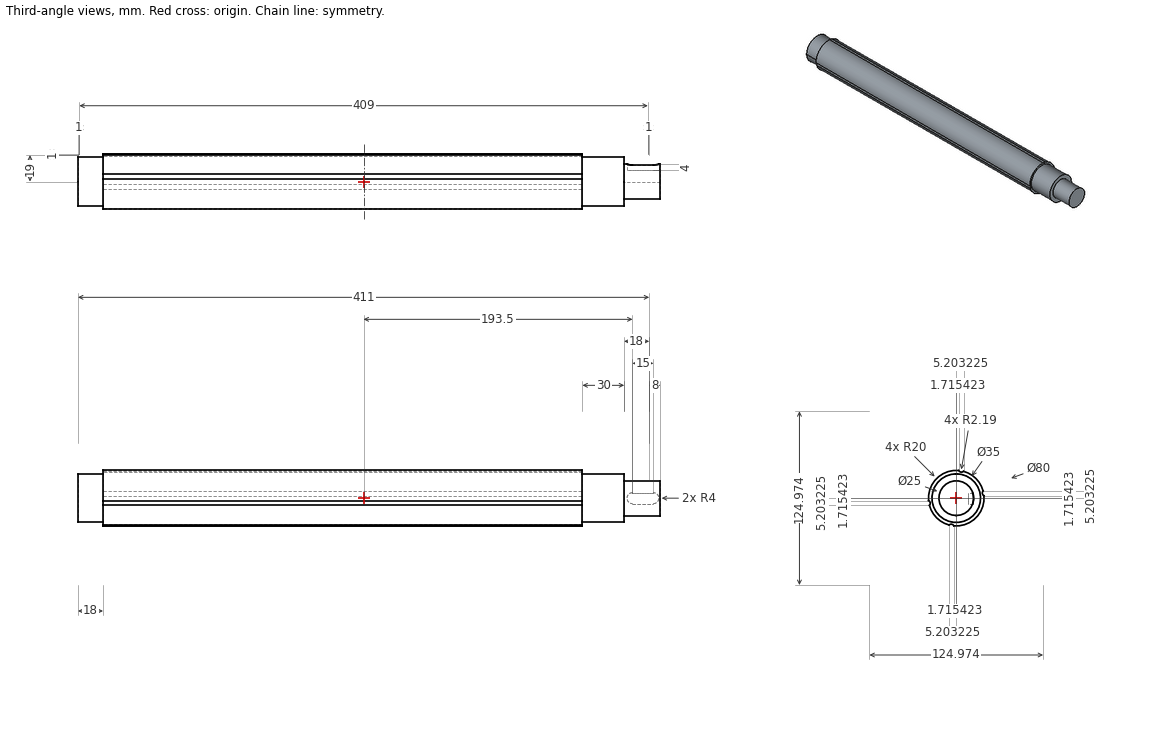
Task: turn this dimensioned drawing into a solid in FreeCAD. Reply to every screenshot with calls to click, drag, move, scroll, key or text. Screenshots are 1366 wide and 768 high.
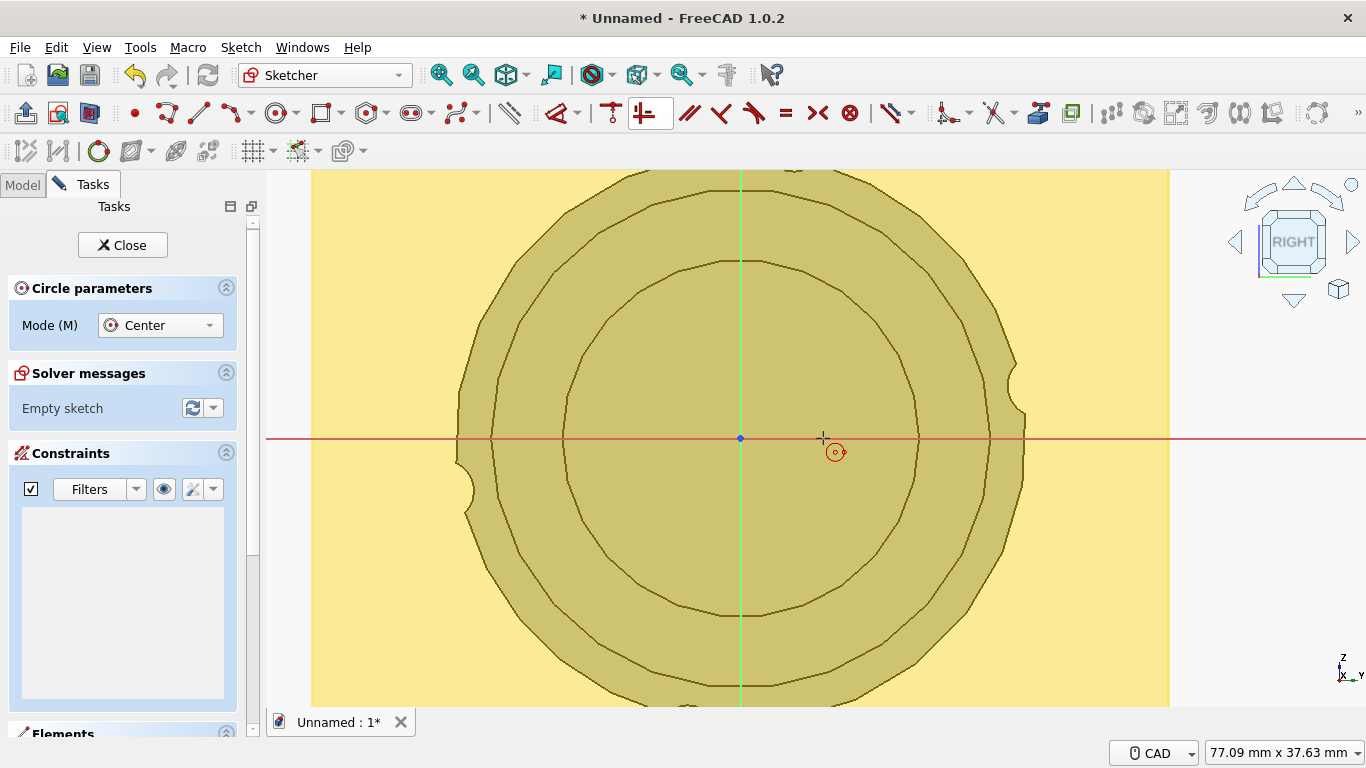
click(741, 438)
click(867, 312)
key(Escape)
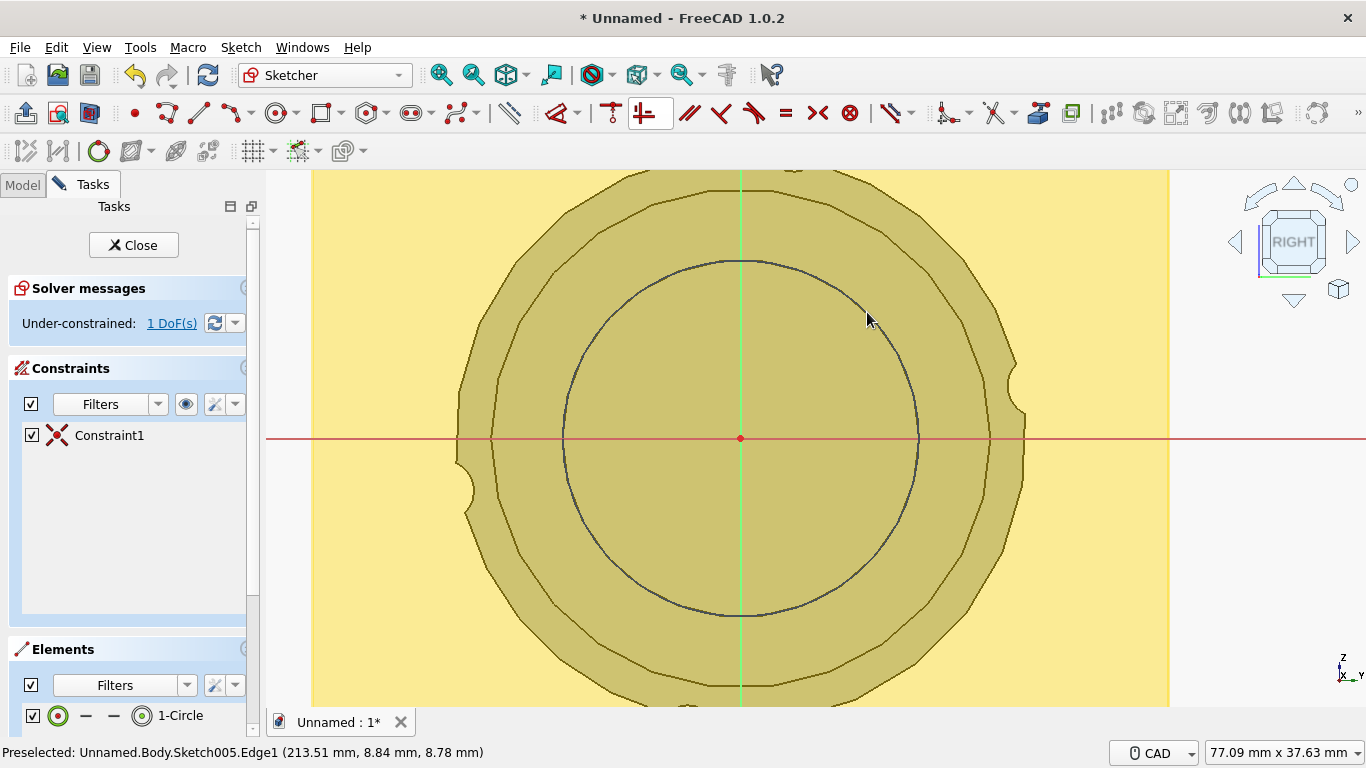
key(d)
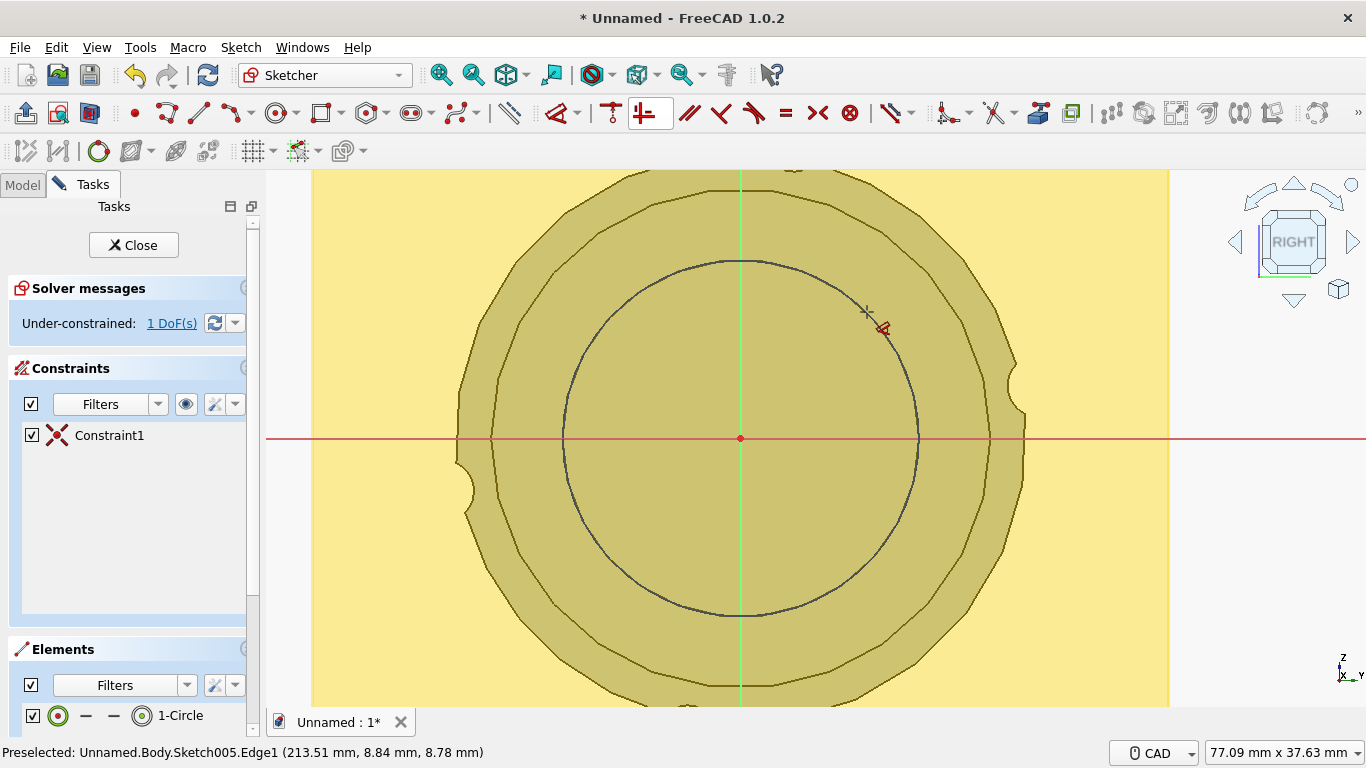
click(866, 312)
click(889, 289)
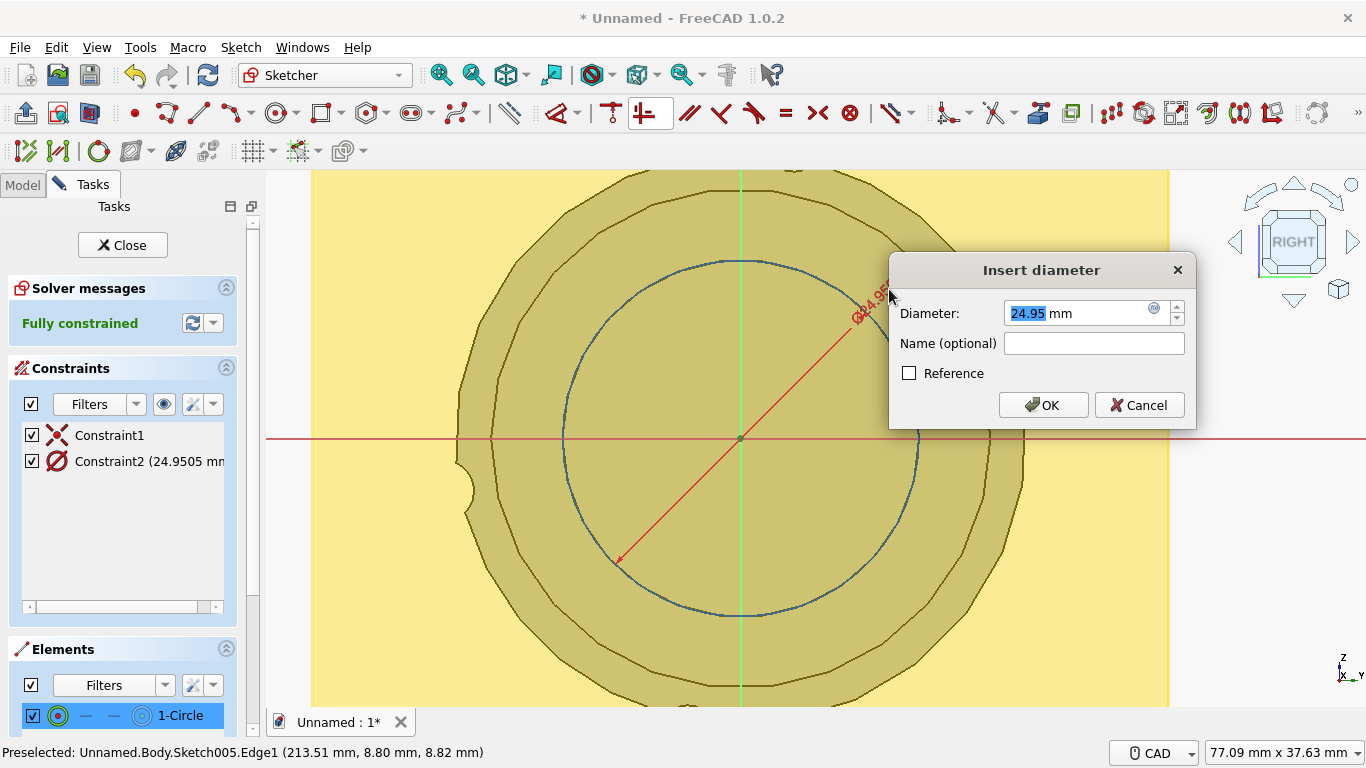
text(25)
key(Return)
key(Escape)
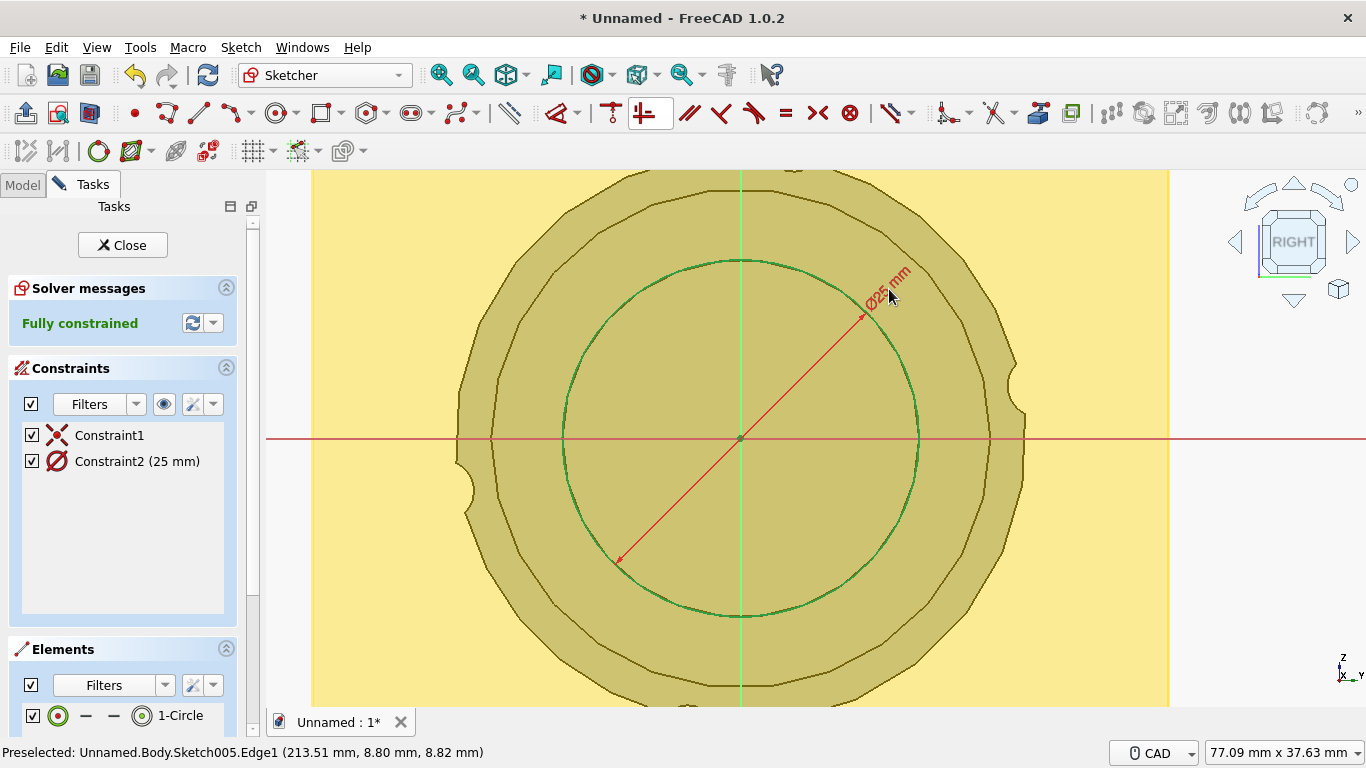
click(123, 245)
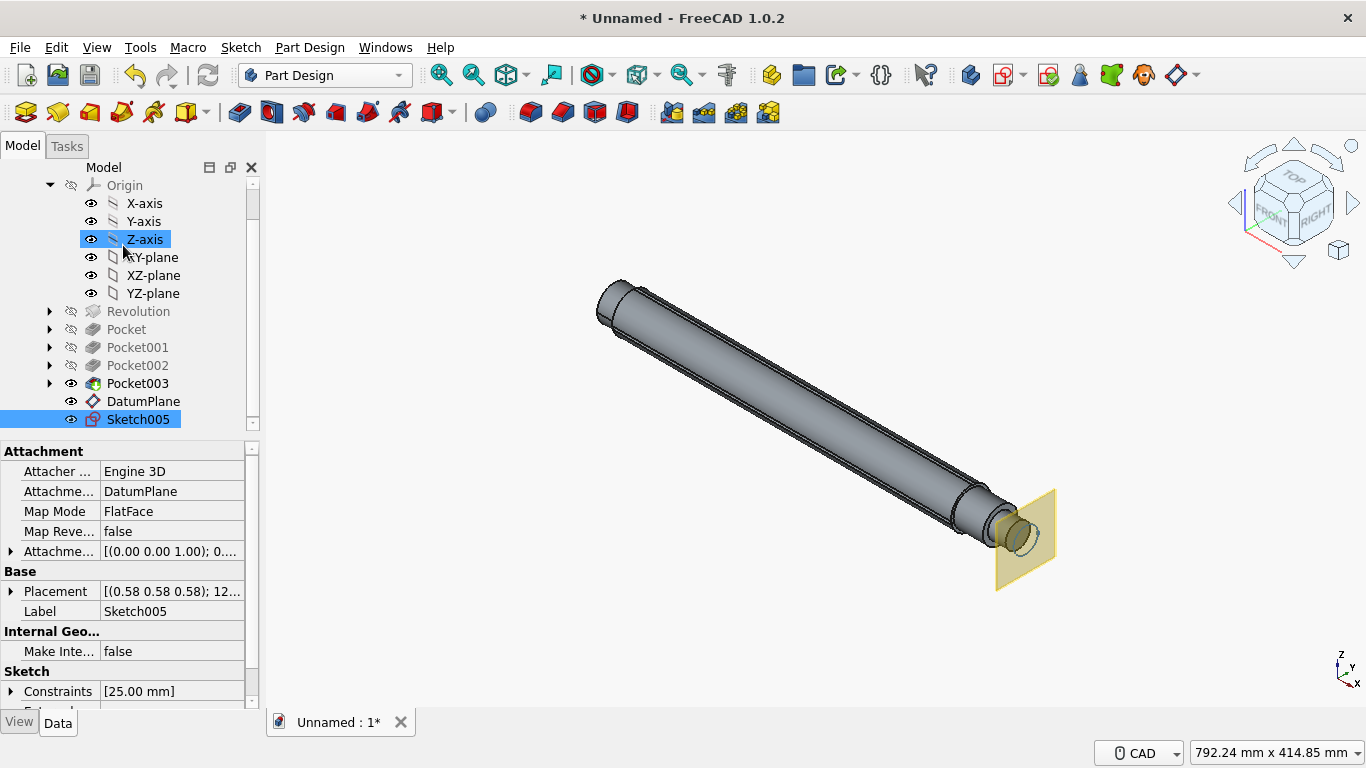
click(26, 112)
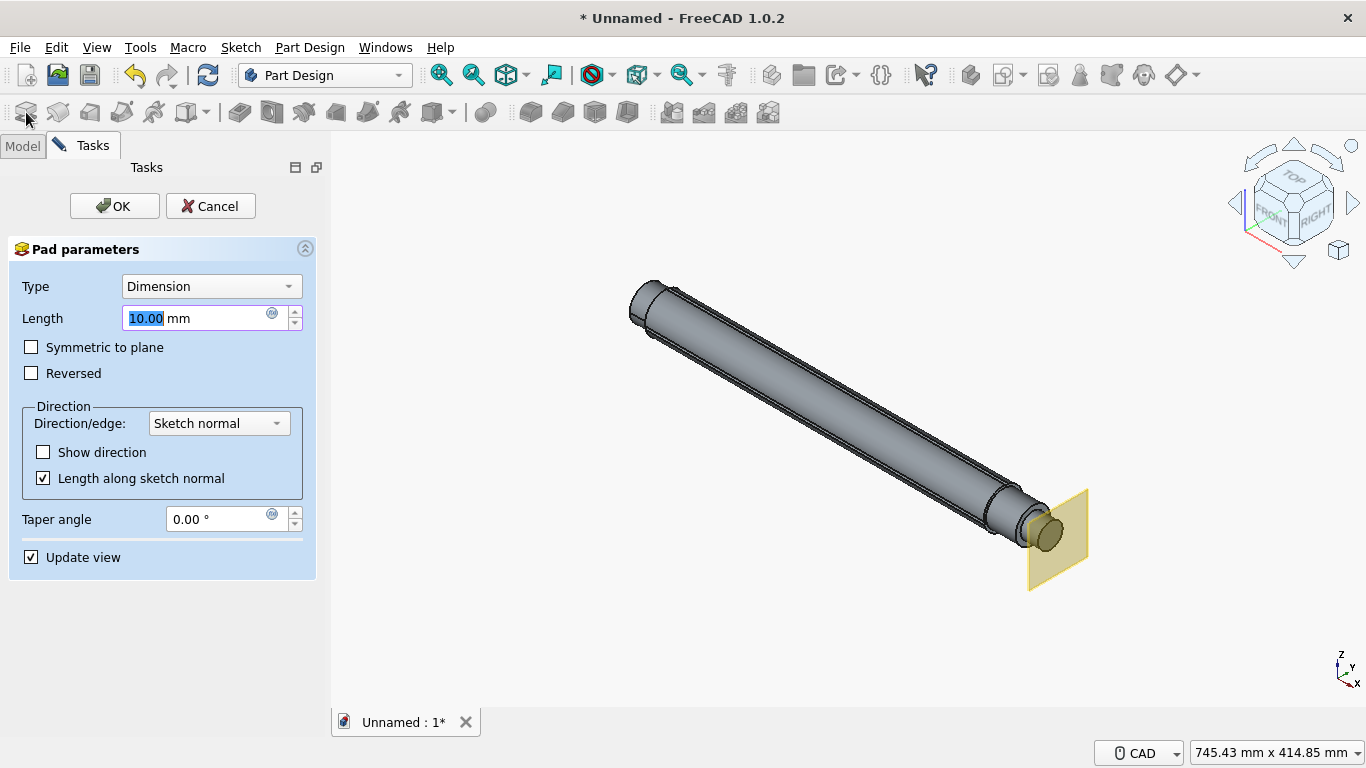
text(8)
key(Tab)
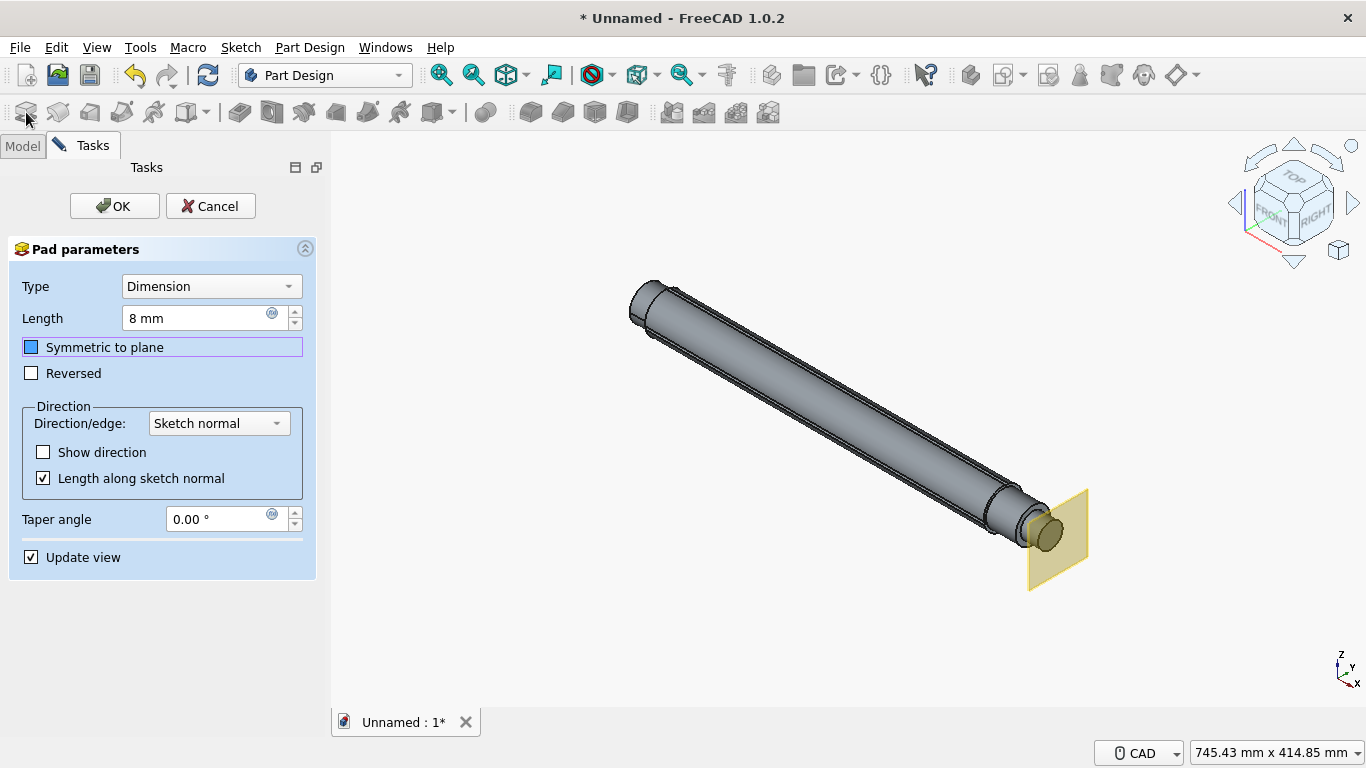
click(30, 373)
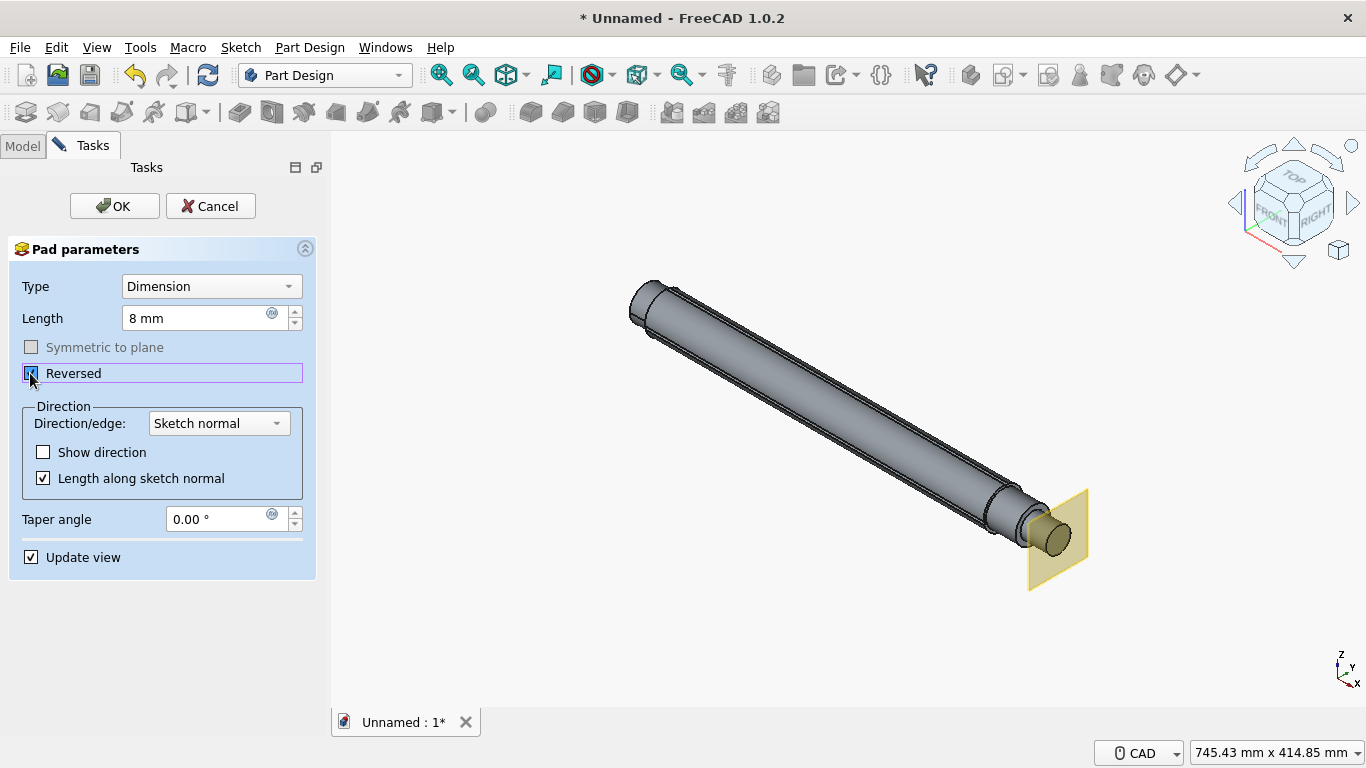
click(115, 206)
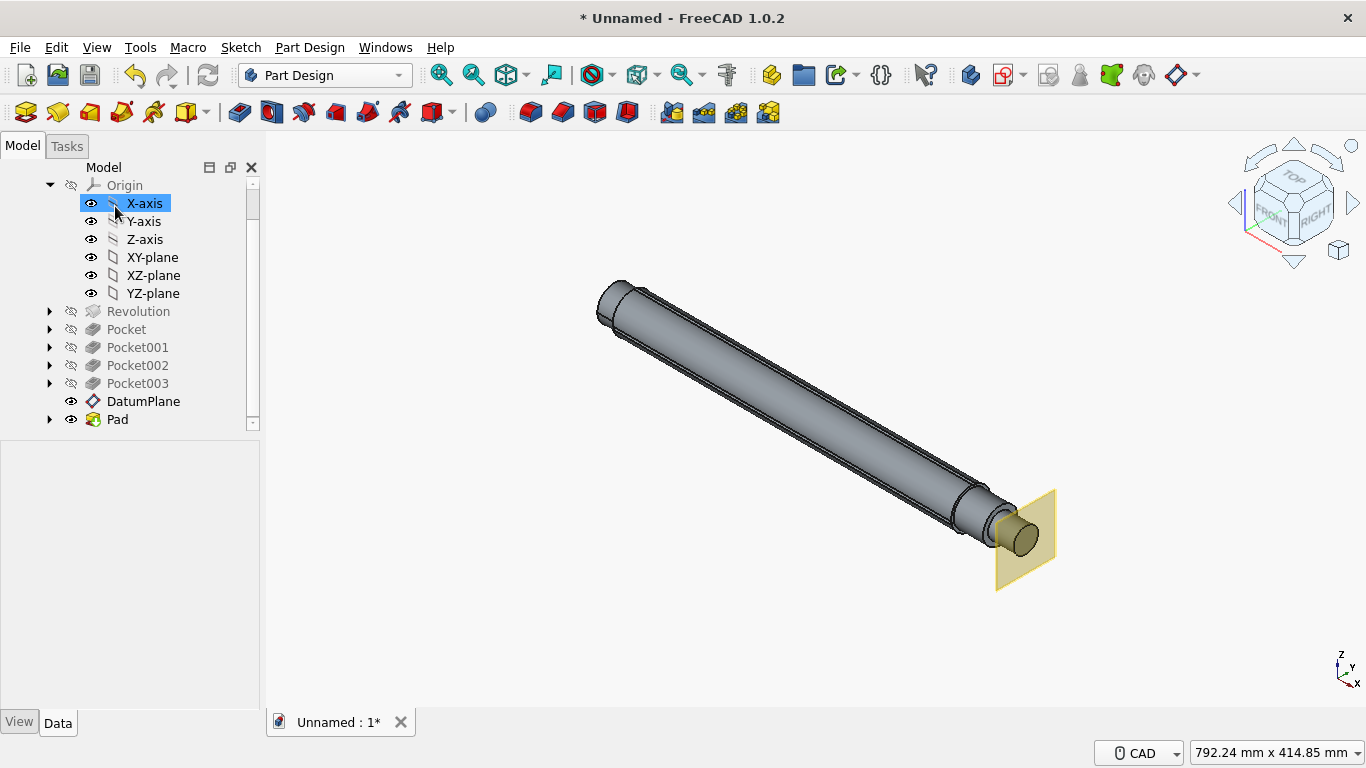
click(116, 401)
key(space)